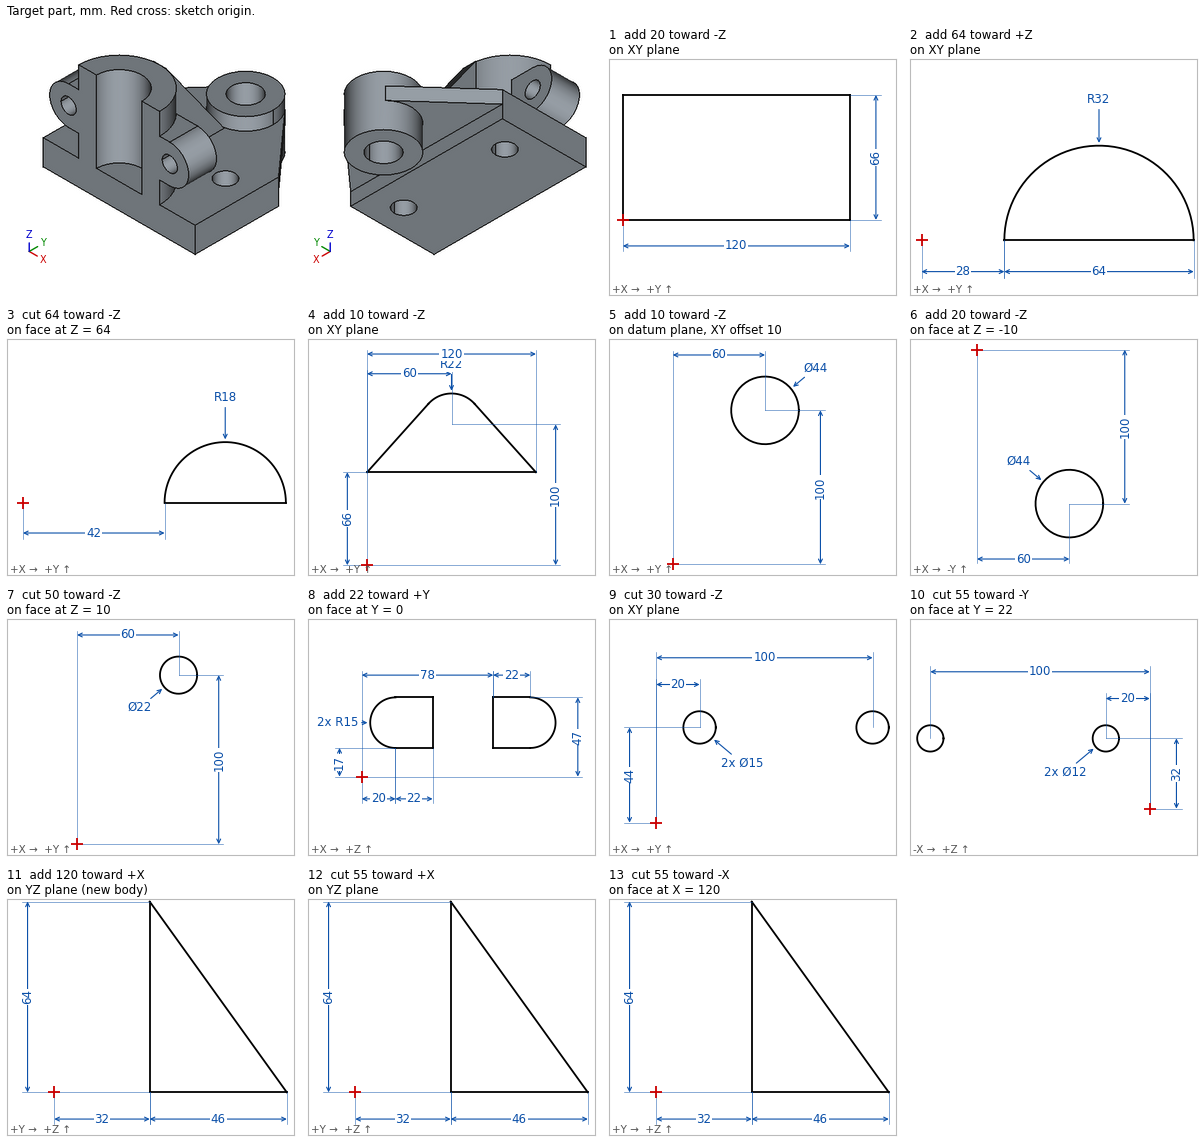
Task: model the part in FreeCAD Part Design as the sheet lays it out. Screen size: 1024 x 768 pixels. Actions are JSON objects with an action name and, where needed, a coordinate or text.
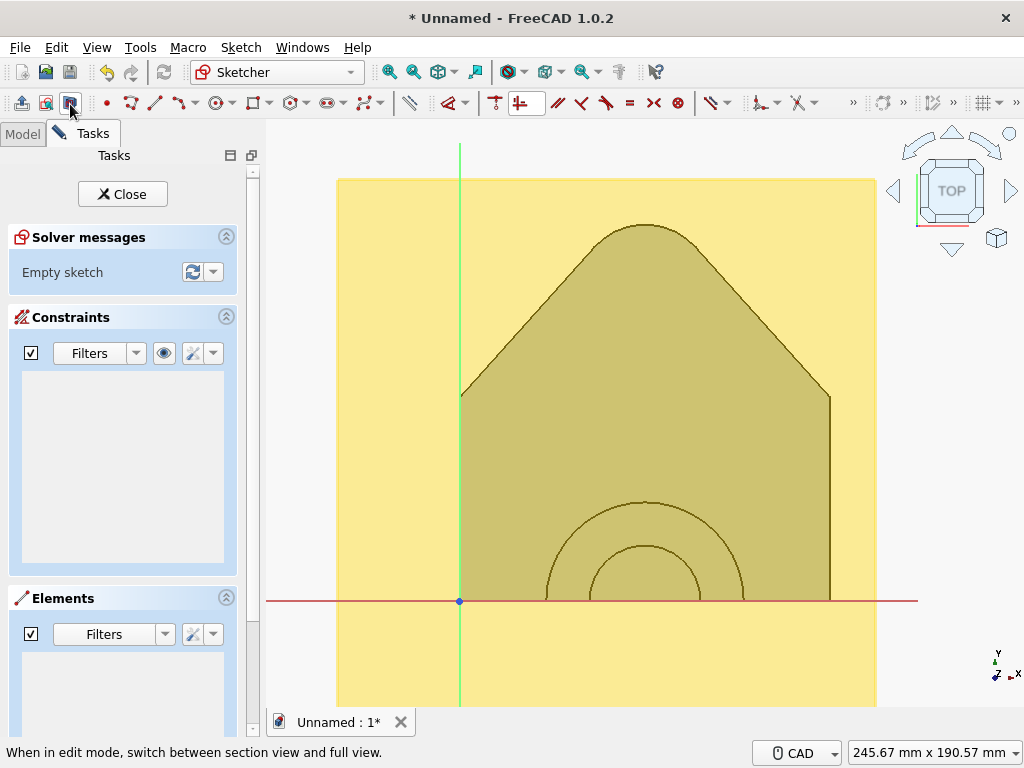
{"action": "scroll", "coordinate": [685, 222], "scroll_direction": "up", "scroll_amount": 5}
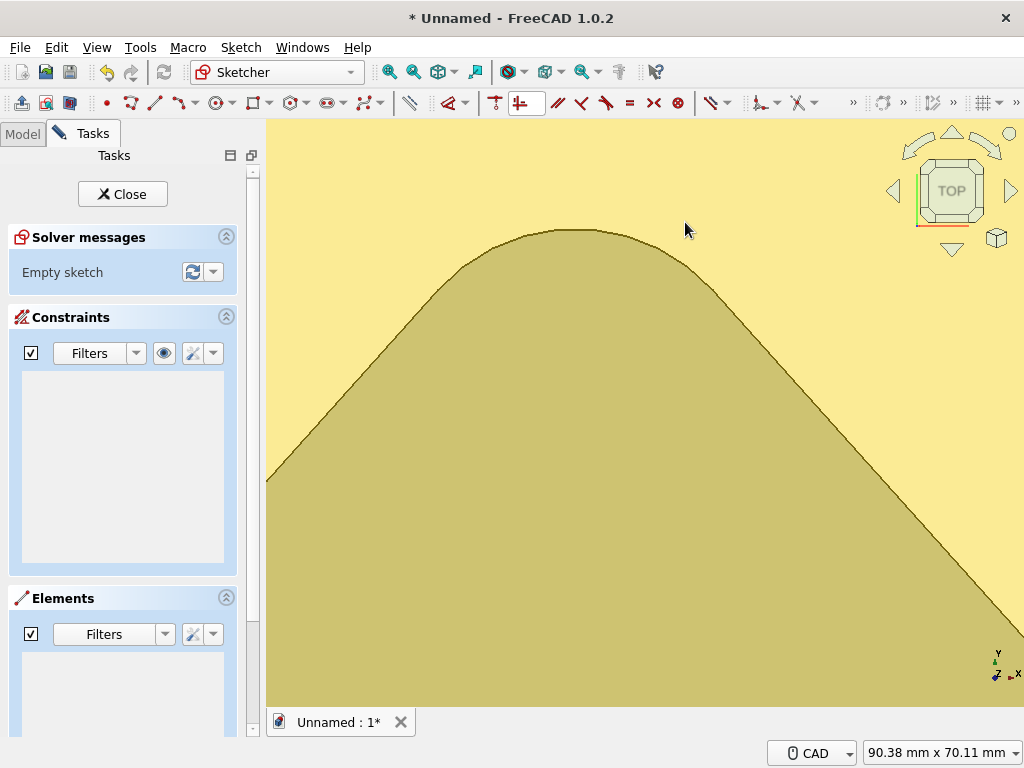
{"action": "left_click", "coordinate": [216, 104]}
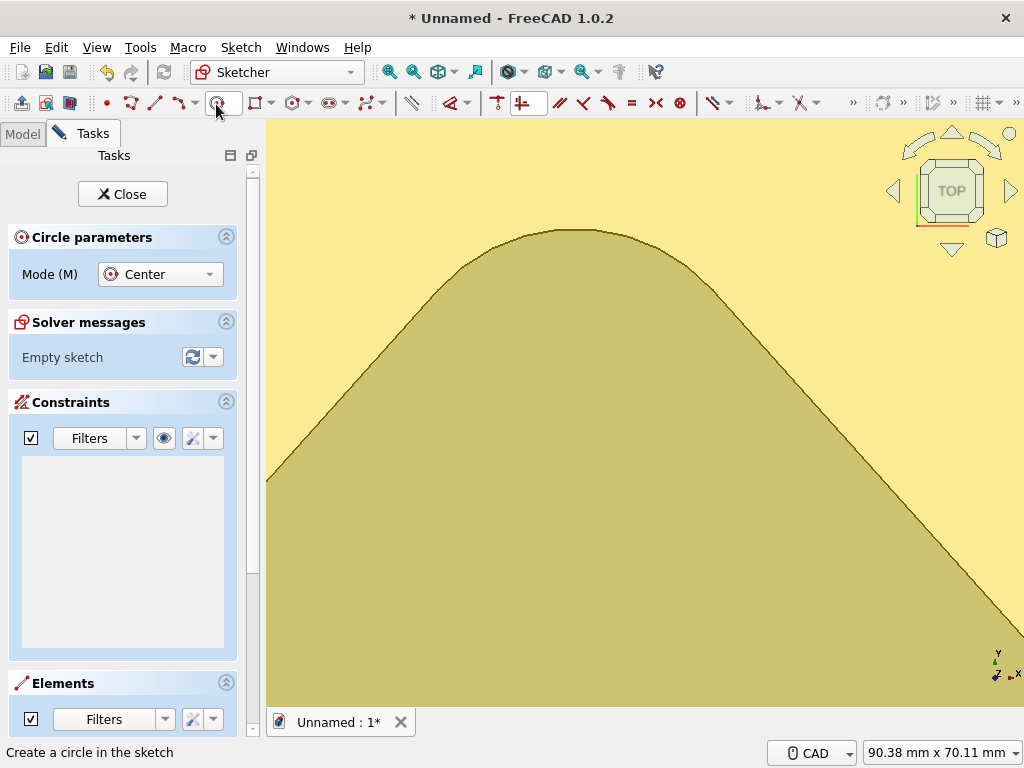
{"action": "left_click", "coordinate": [575, 413]}
{"action": "left_click", "coordinate": [706, 283]}
{"action": "key", "text": "Escape"}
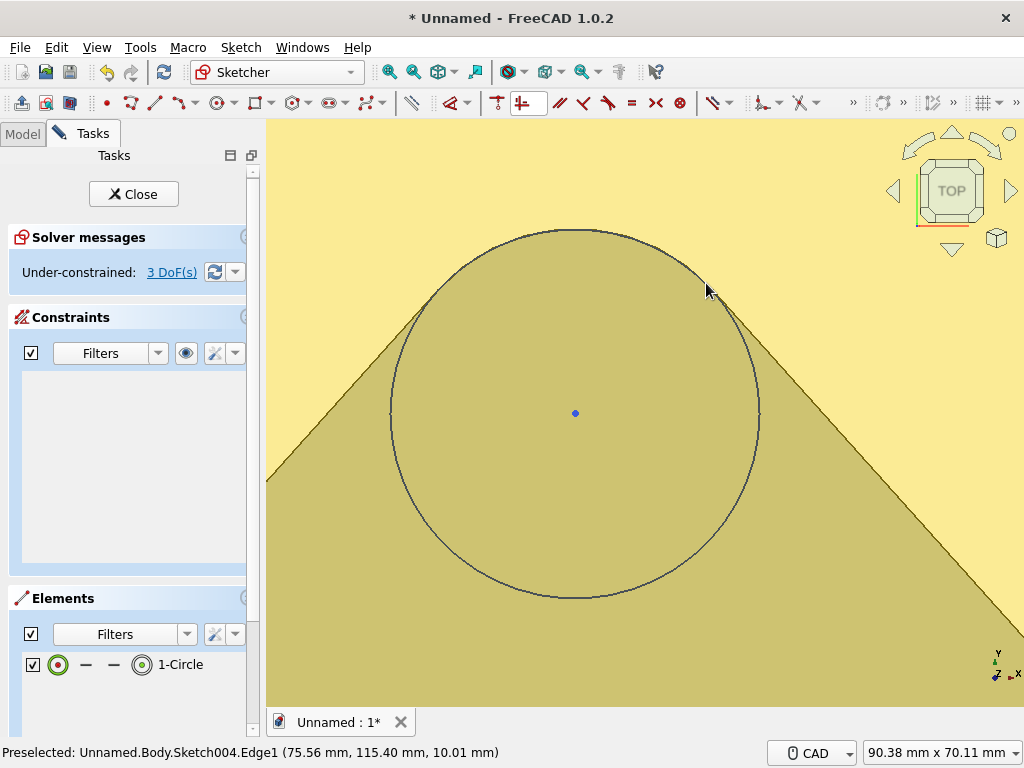
{"action": "left_click", "coordinate": [450, 104]}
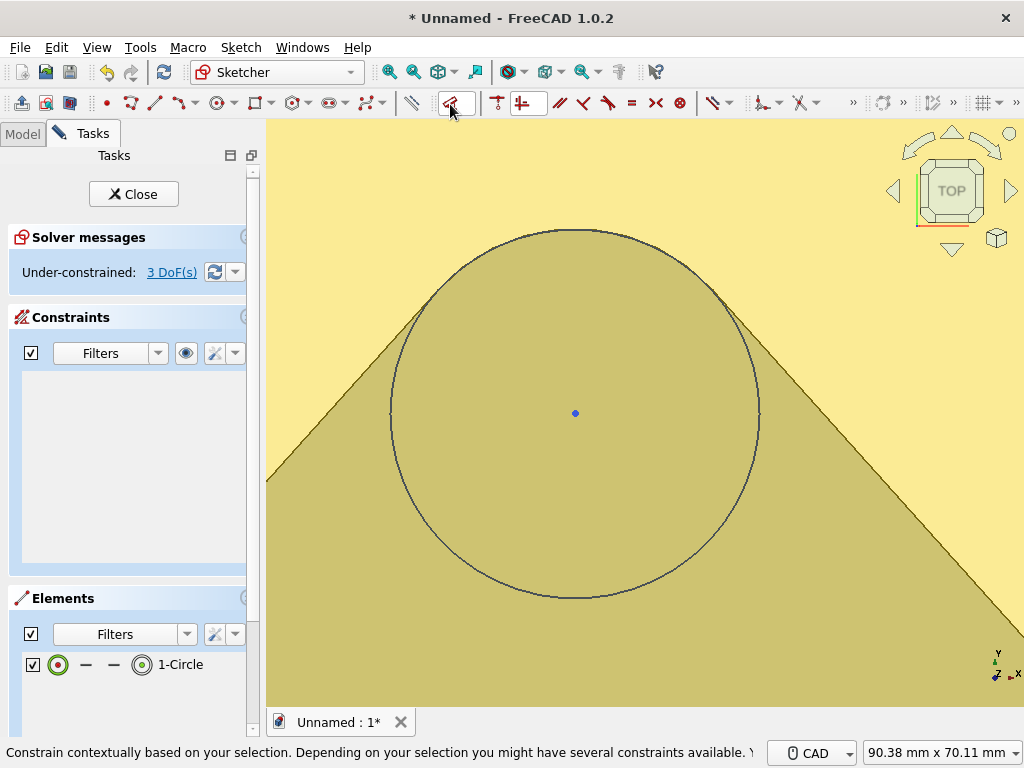
{"action": "left_click", "coordinate": [705, 283]}
{"action": "left_click", "coordinate": [728, 260]}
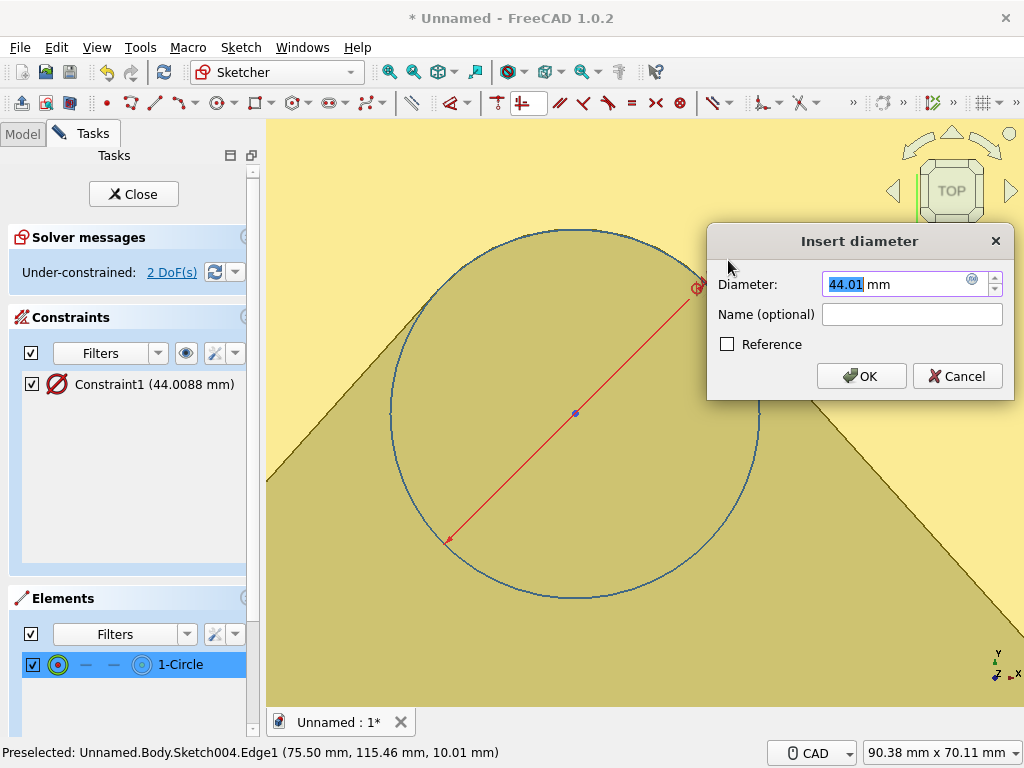
{"action": "type", "text": "44"}
{"action": "key", "text": "Return"}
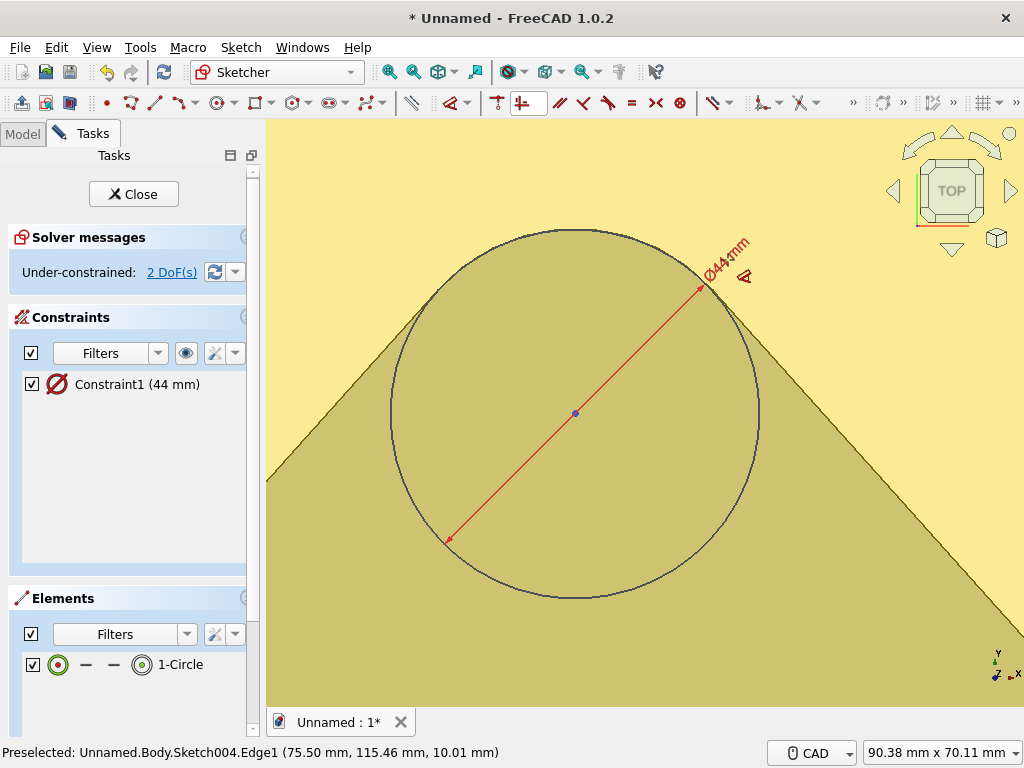
{"action": "left_click", "coordinate": [575, 414]}
{"action": "left_click", "coordinate": [435, 380]}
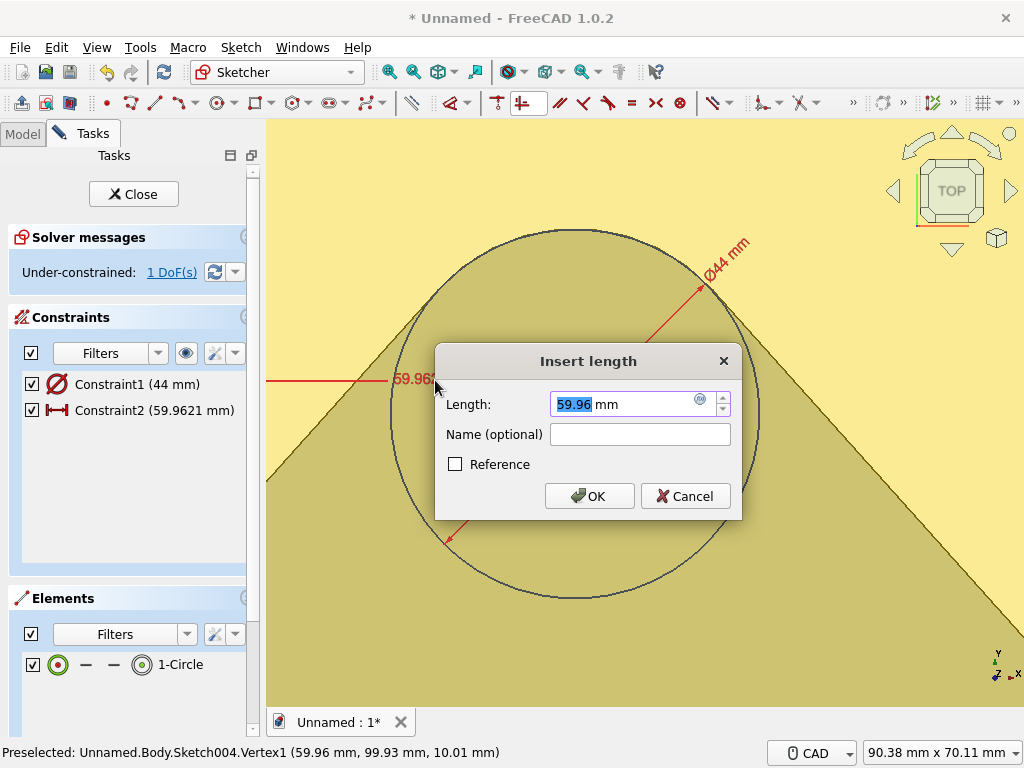
{"action": "type", "text": "60"}
{"action": "key", "text": "Return"}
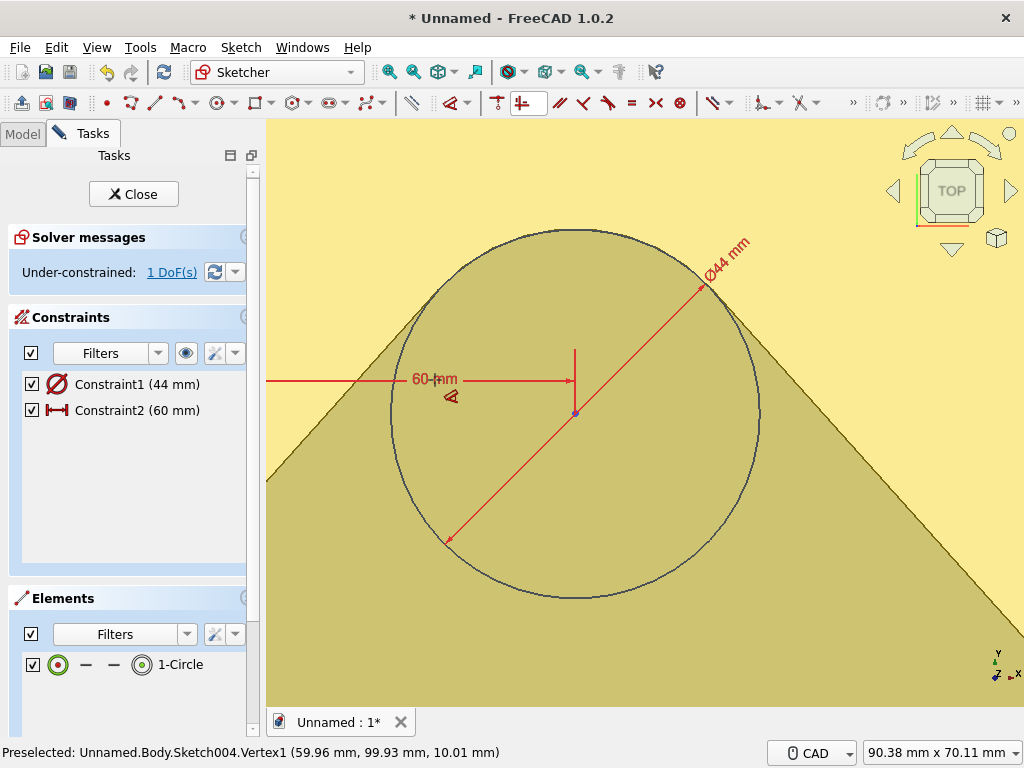
{"action": "left_click", "coordinate": [575, 414]}
{"action": "left_click", "coordinate": [609, 546]}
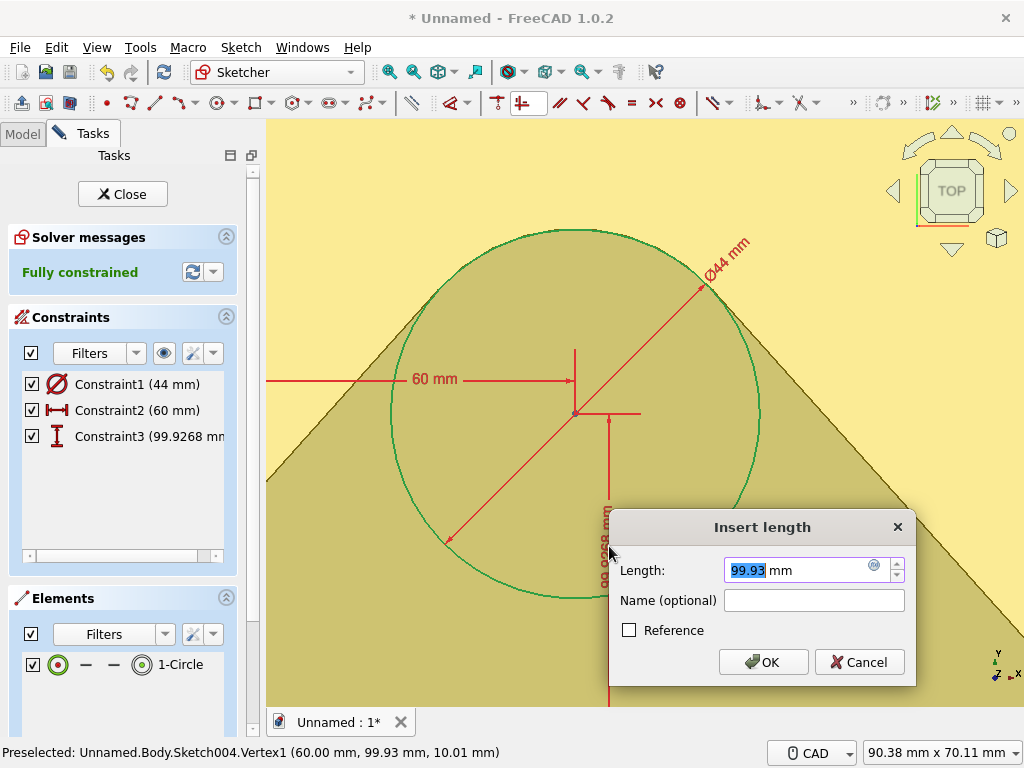
{"action": "type", "text": "100"}
{"action": "key", "text": "Return"}
{"action": "key", "text": "Escape"}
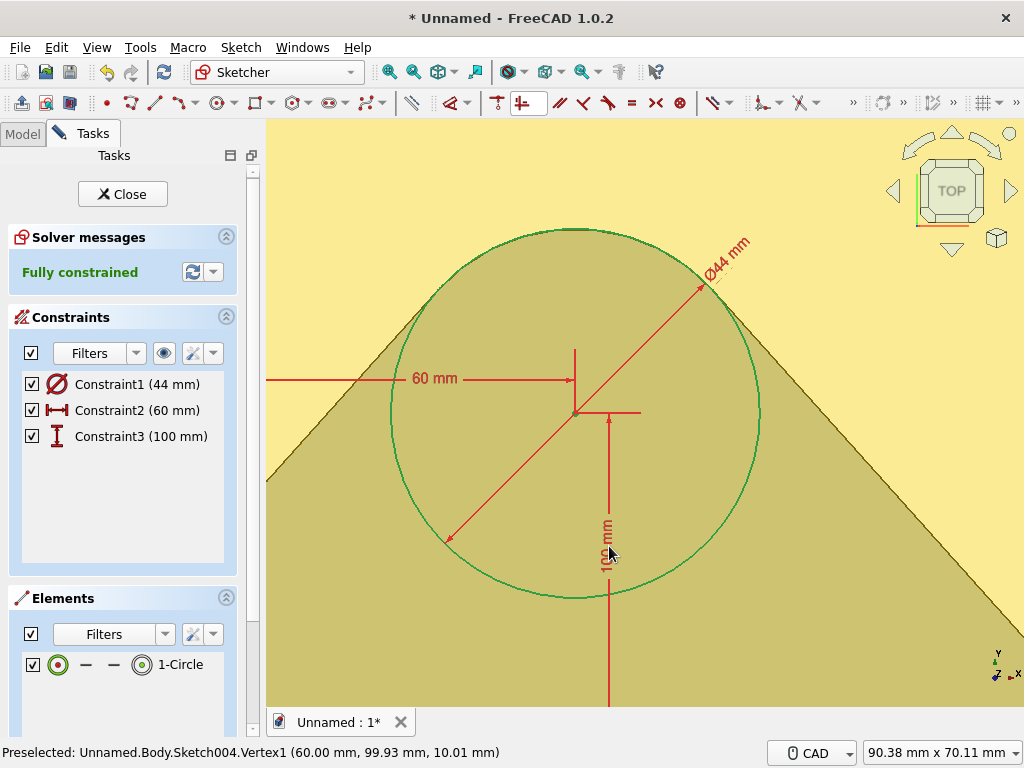
{"action": "left_click", "coordinate": [123, 194]}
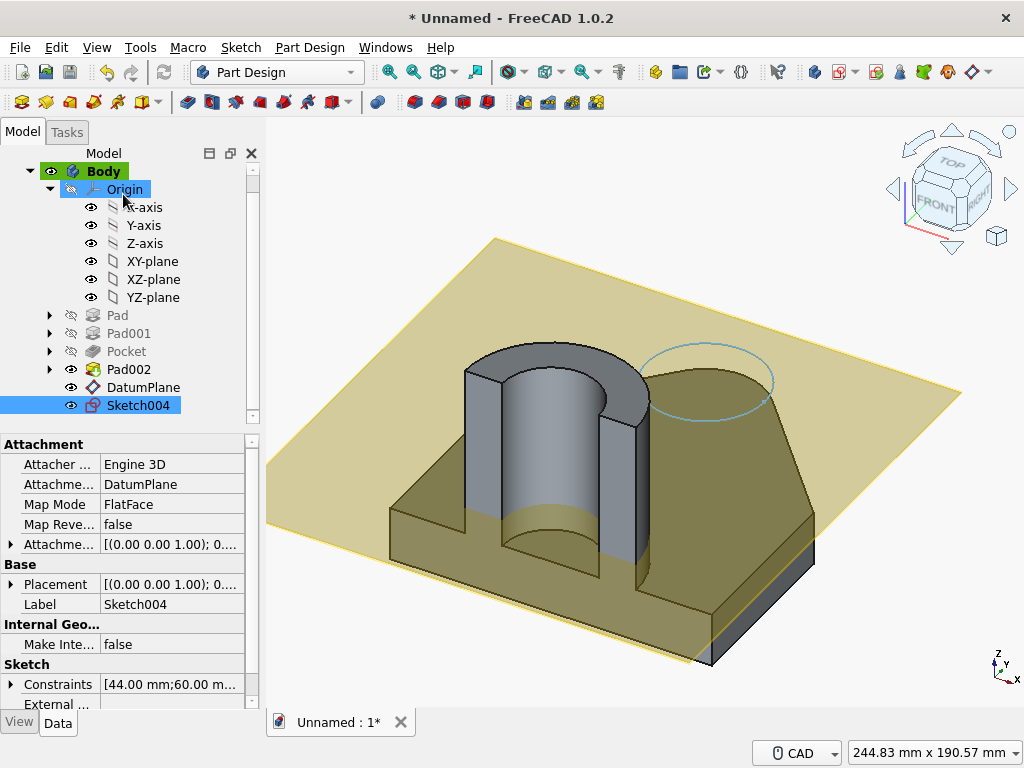
{"action": "left_click", "coordinate": [22, 102]}